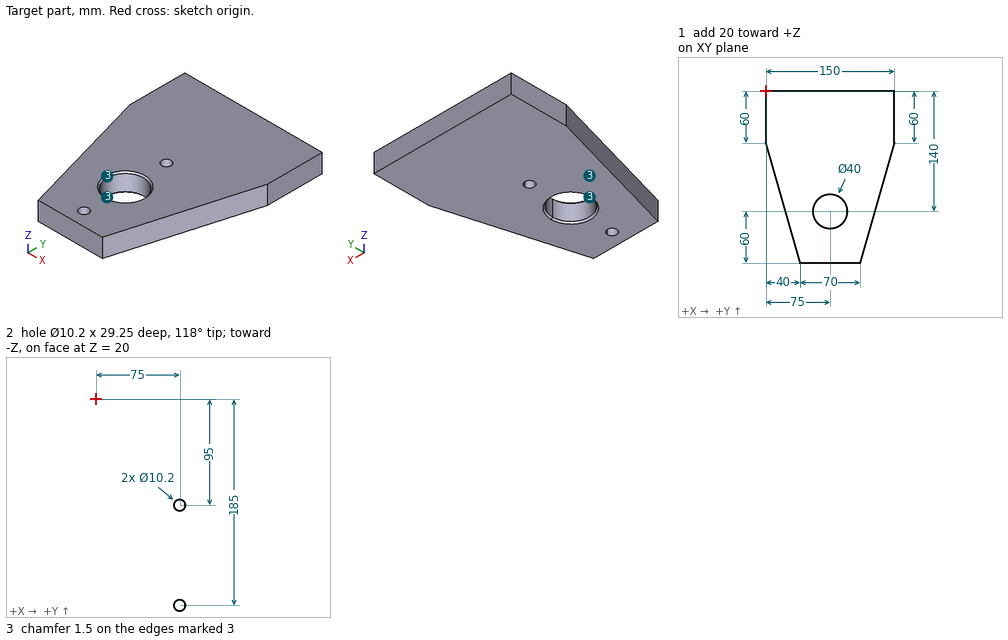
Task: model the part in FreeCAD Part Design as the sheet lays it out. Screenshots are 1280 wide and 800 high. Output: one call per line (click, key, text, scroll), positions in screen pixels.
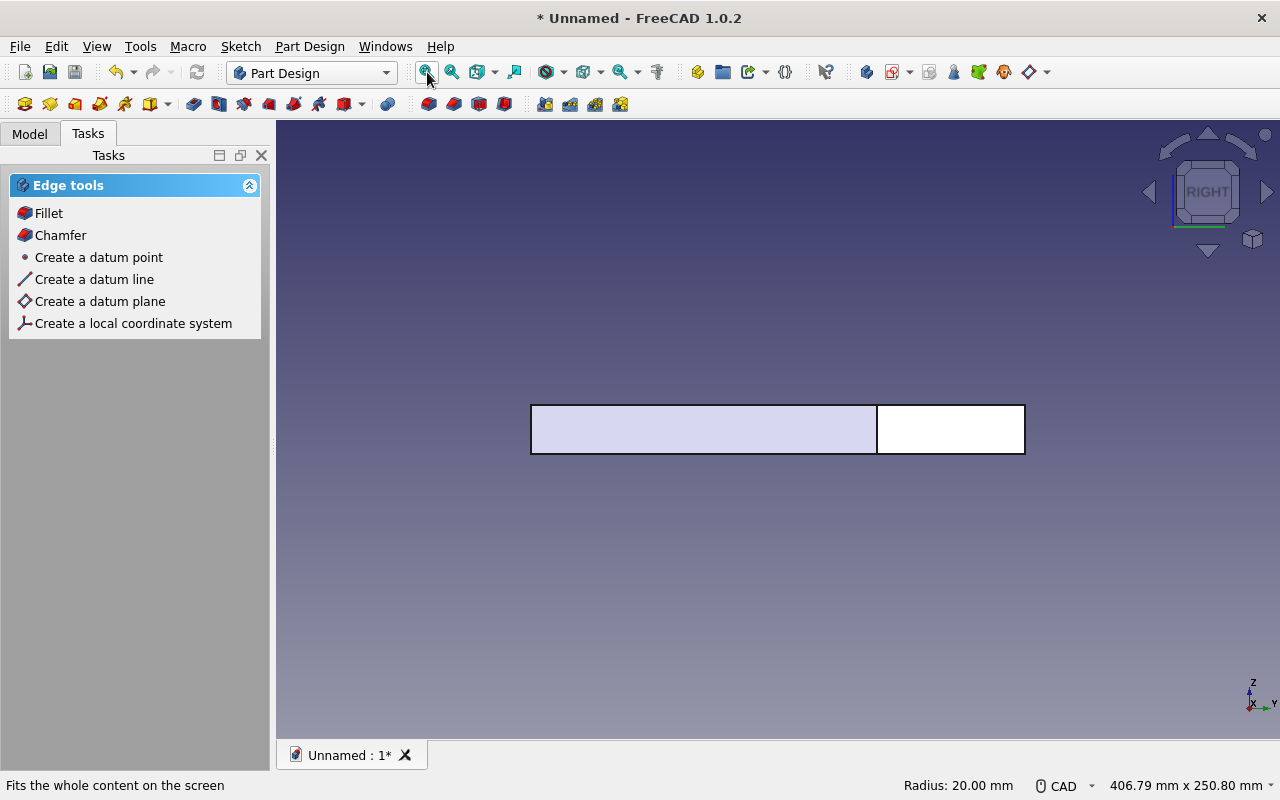
key(5)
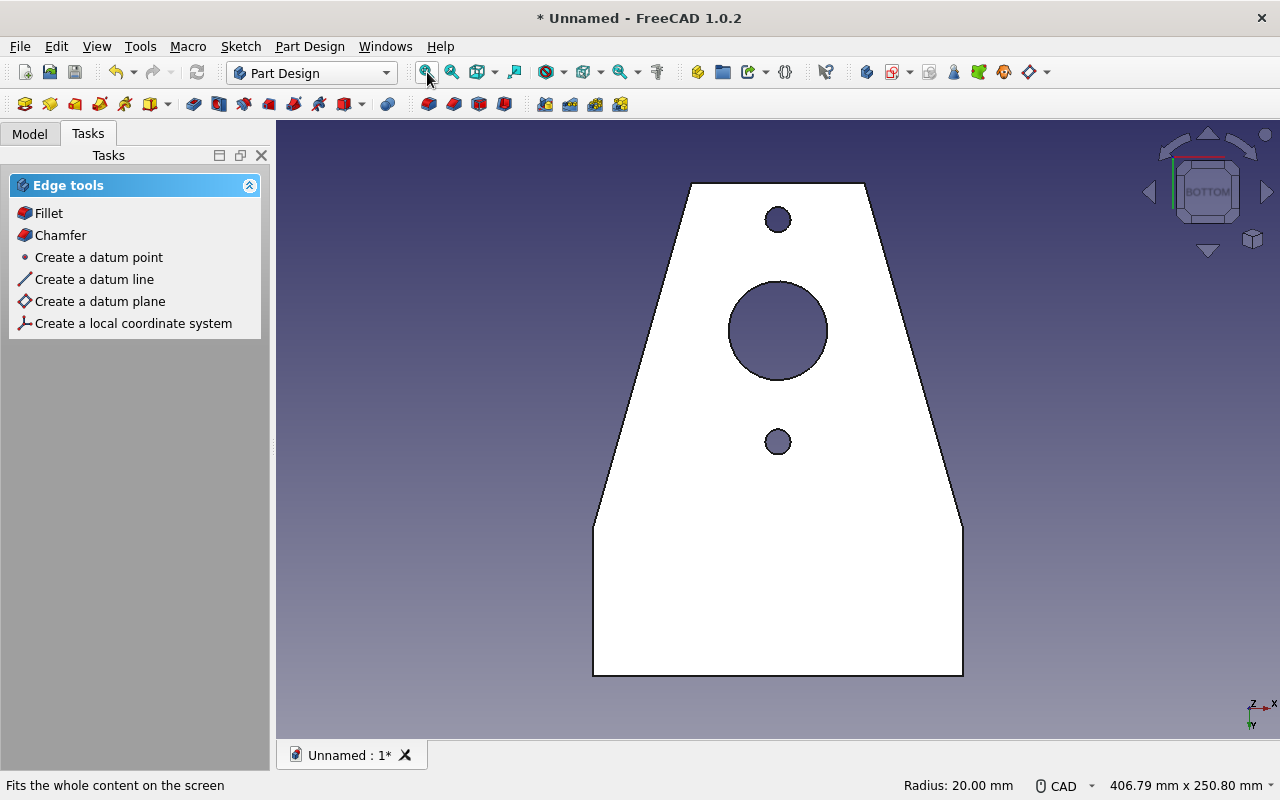
click(729, 330, ctrl)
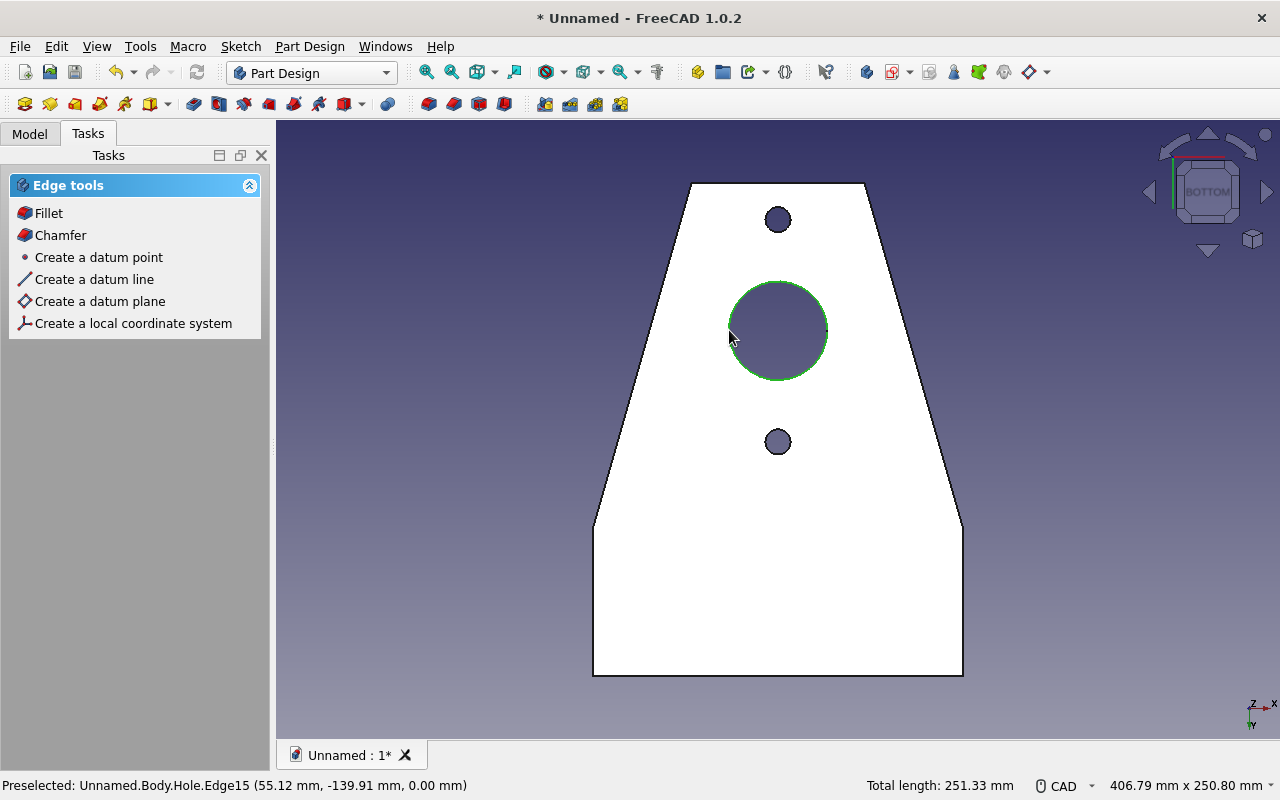
click(454, 104)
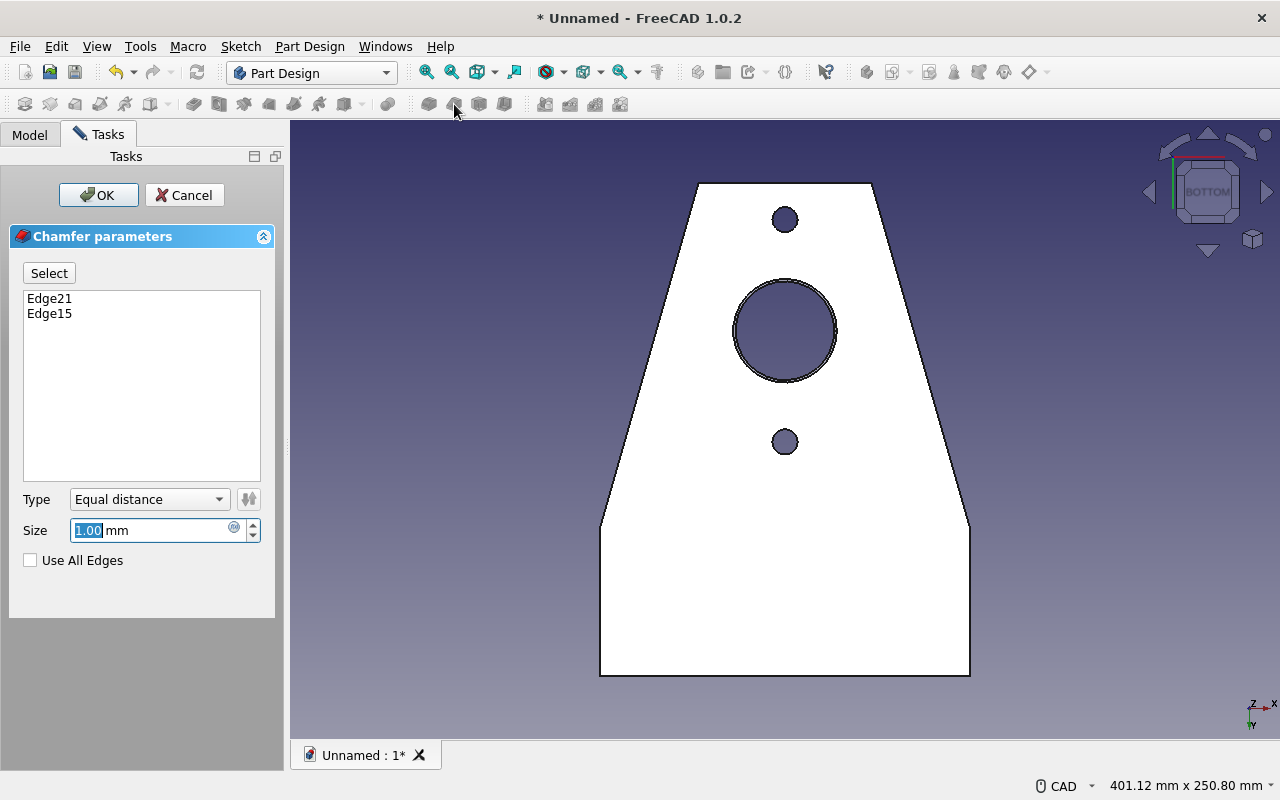
text(1.5)
key(Tab)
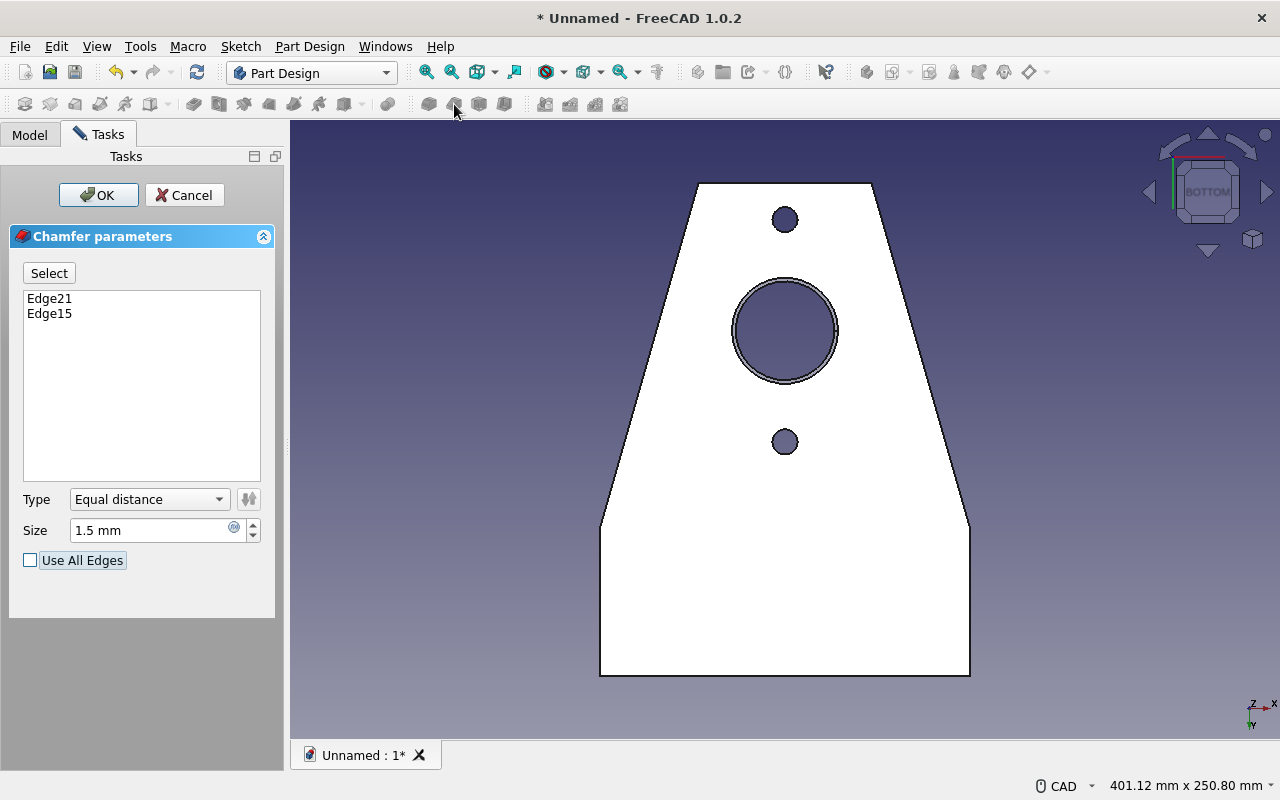
click(99, 195)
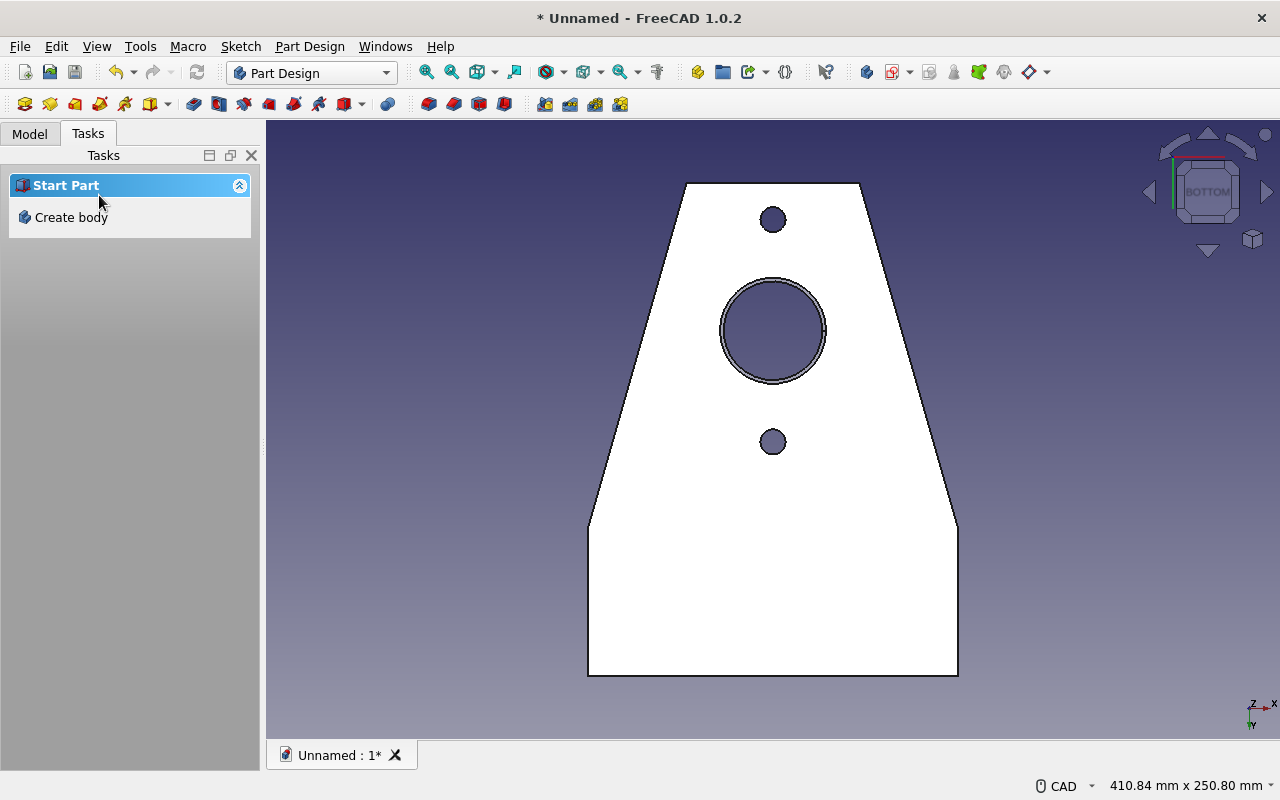
key(0)